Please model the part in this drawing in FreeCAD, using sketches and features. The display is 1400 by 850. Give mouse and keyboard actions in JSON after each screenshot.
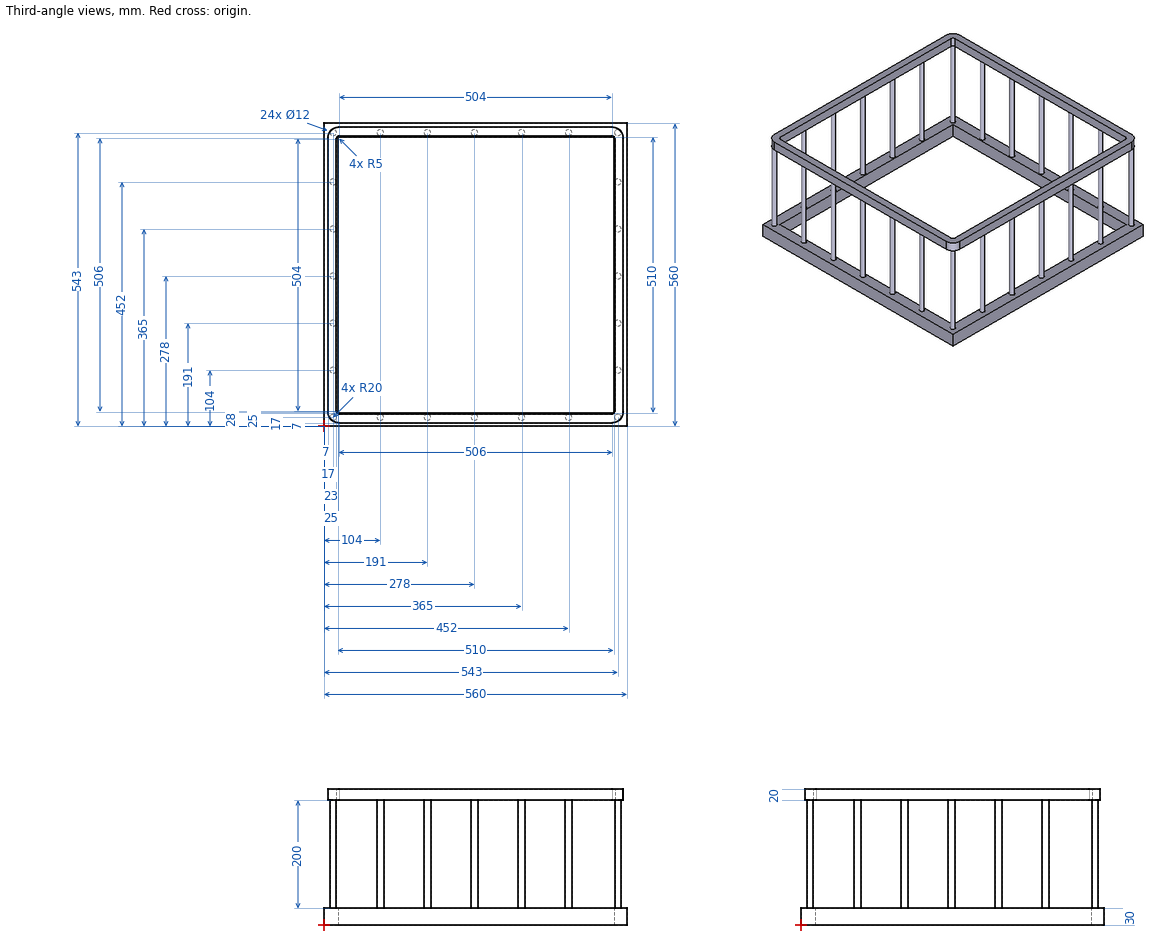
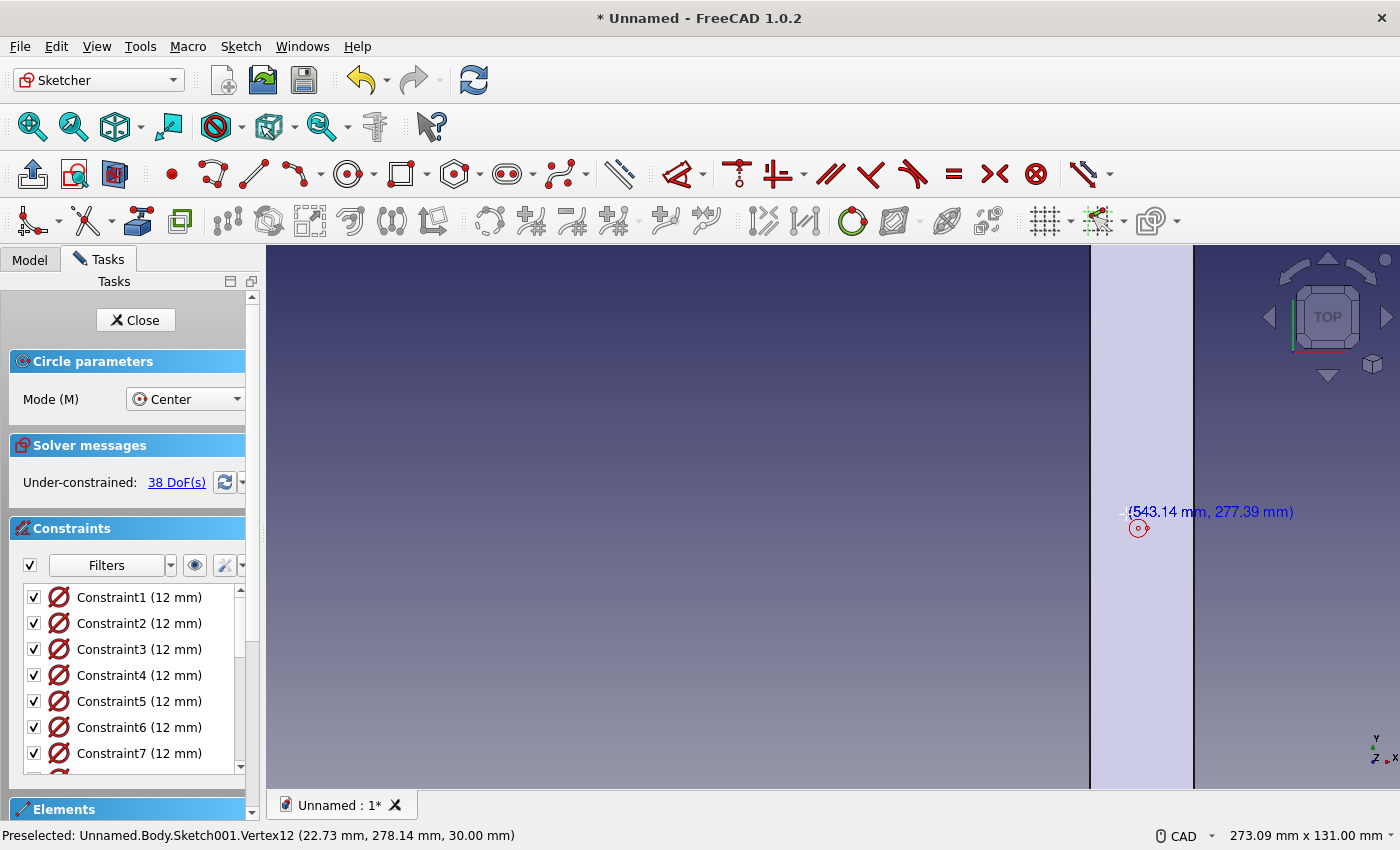
{"action": "scroll", "coordinate": [914, 515], "scroll_direction": "down", "scroll_amount": 9}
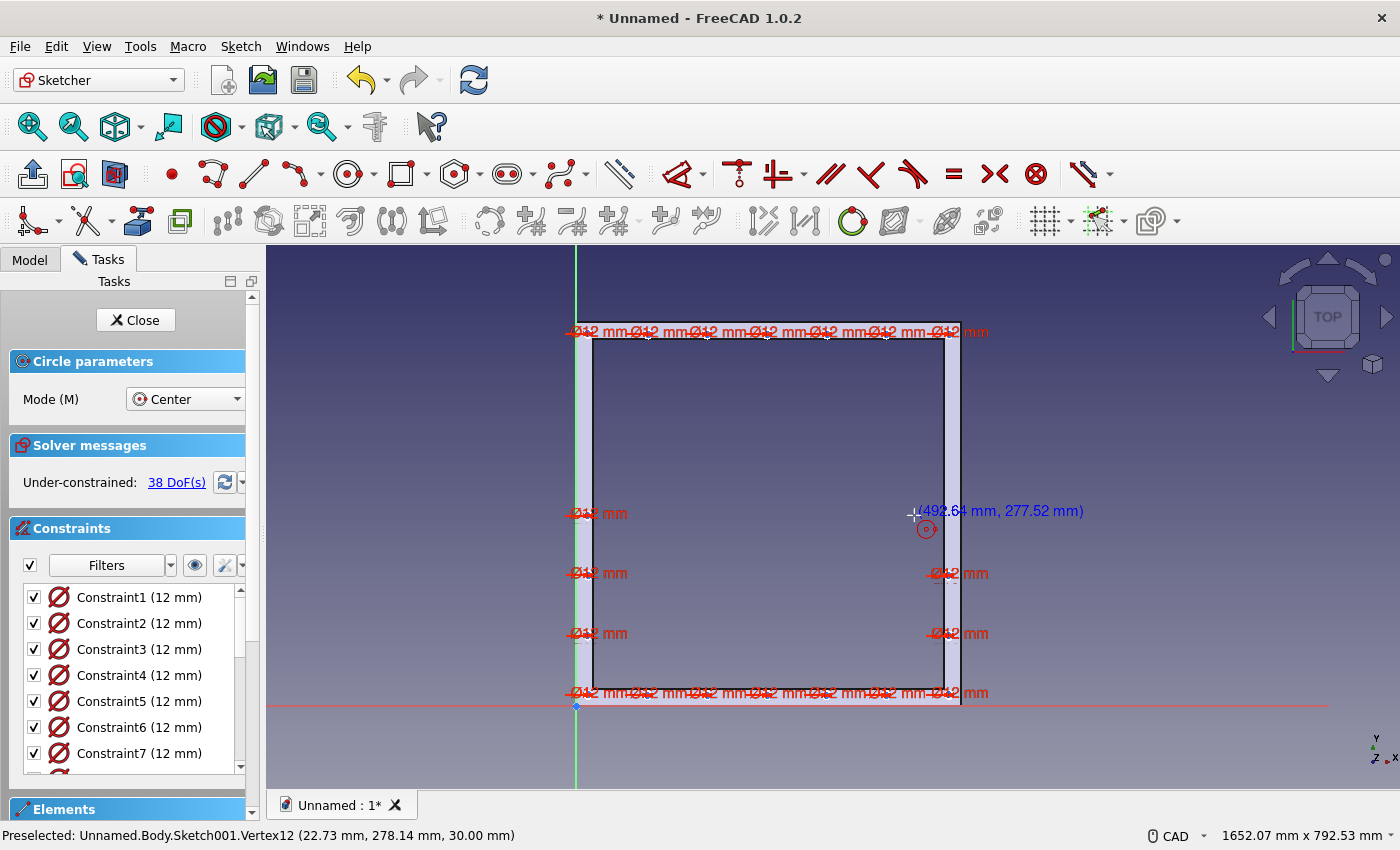
{"action": "left_click", "coordinate": [949, 515]}
{"action": "mouse_move", "coordinate": [952, 512]}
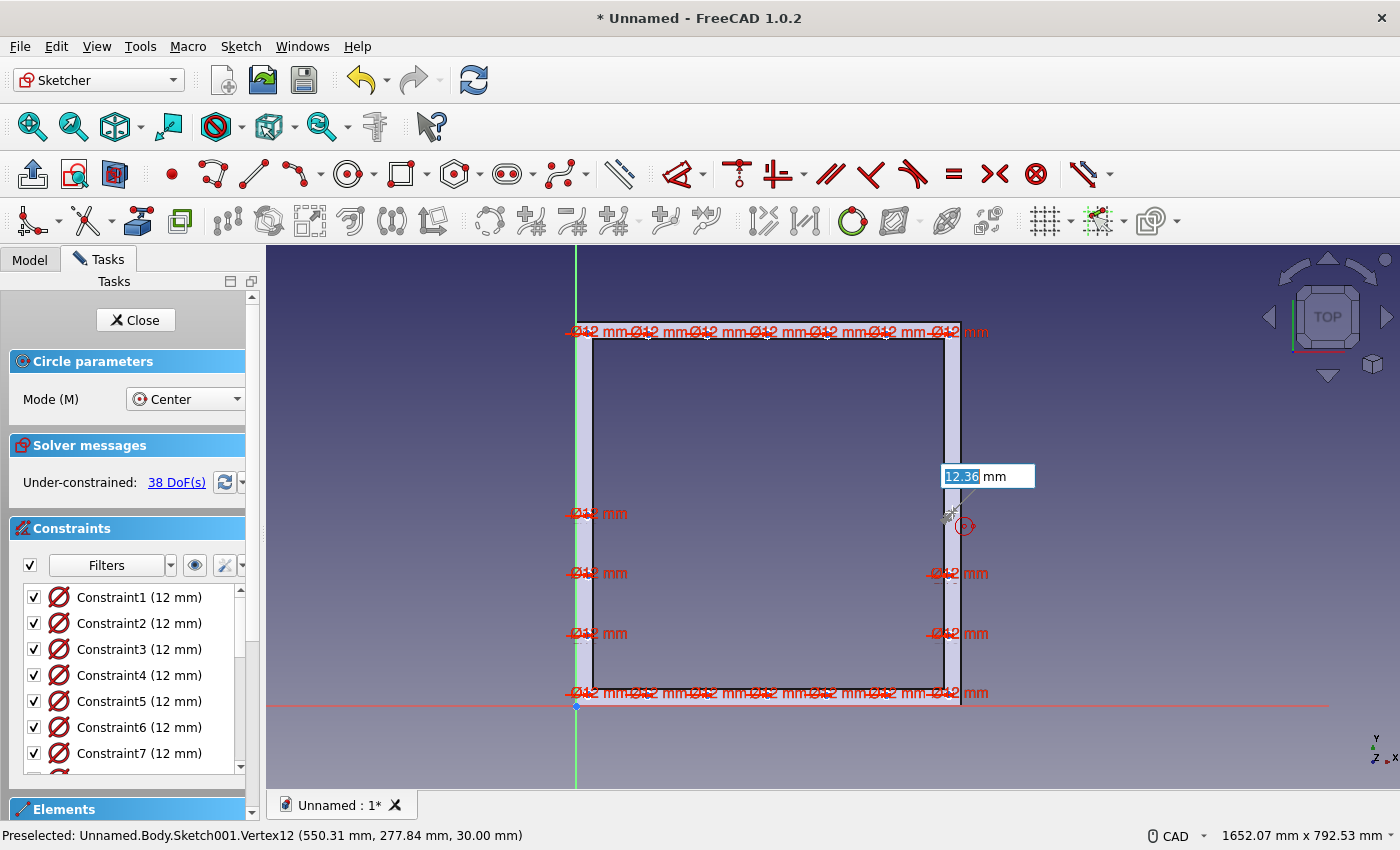
{"action": "type", "text": "12"}
{"action": "key", "text": "Return"}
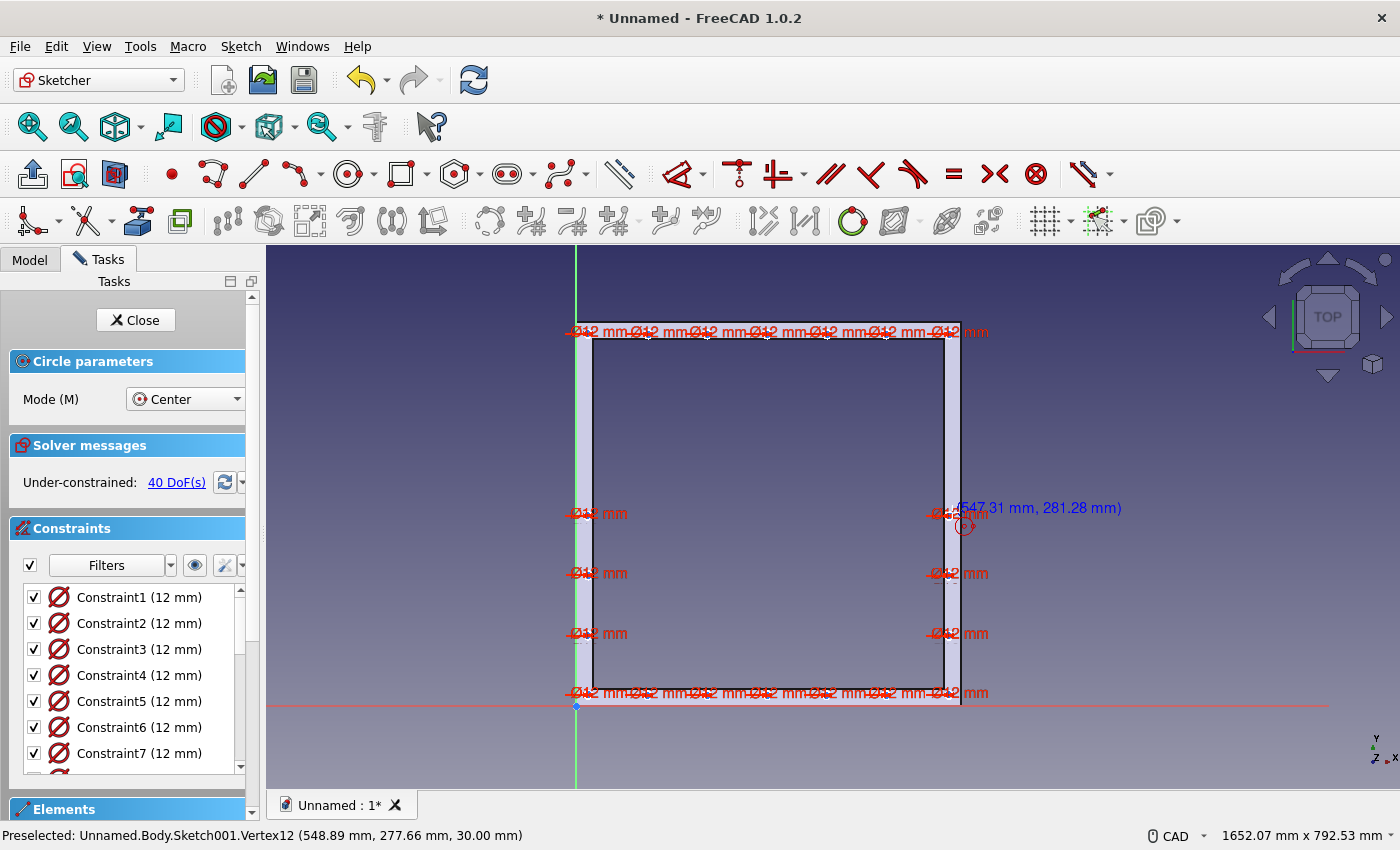
{"action": "scroll", "coordinate": [588, 456], "scroll_direction": "up", "scroll_amount": 9}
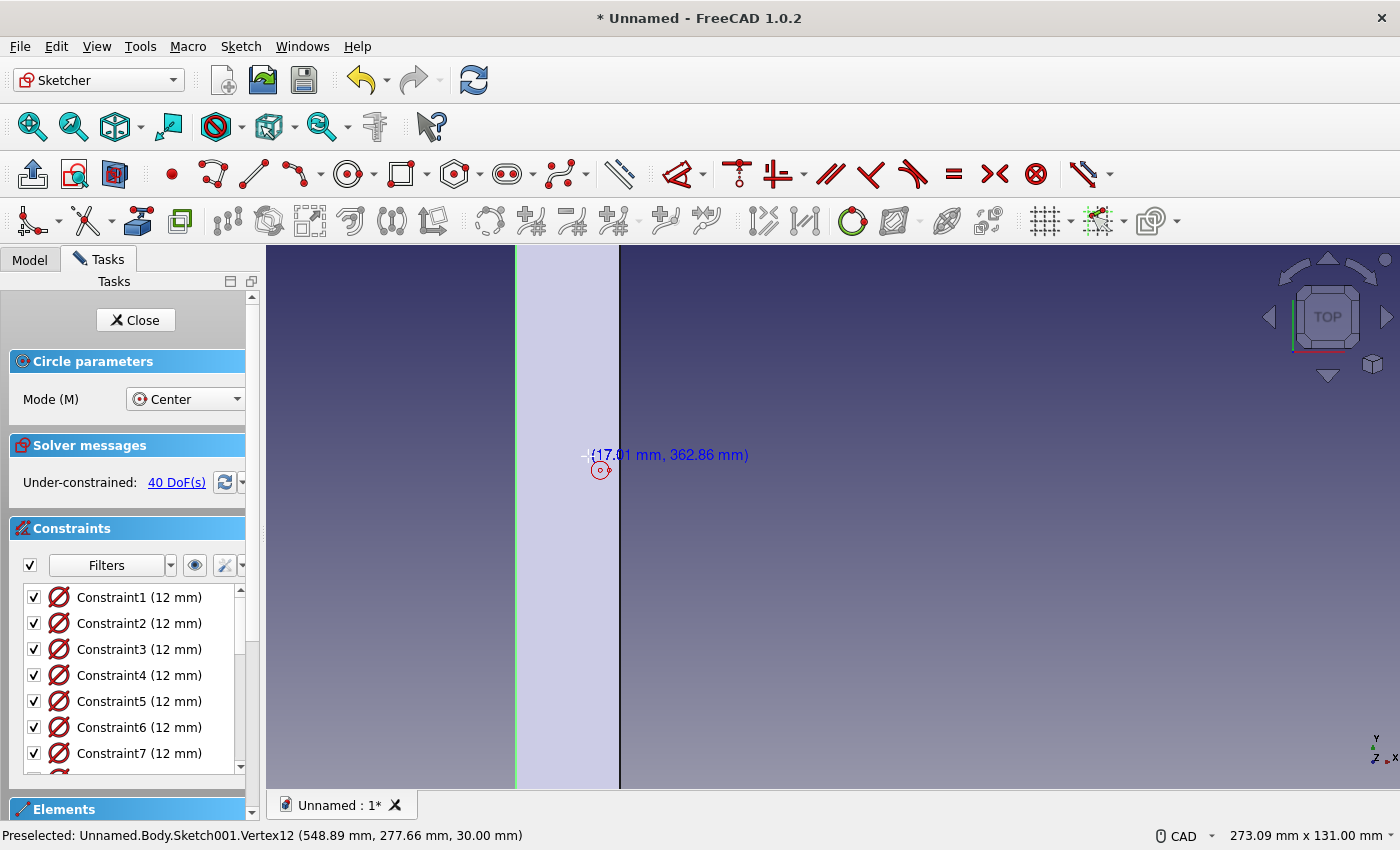
{"action": "scroll", "coordinate": [588, 456], "scroll_direction": "down", "scroll_amount": 9}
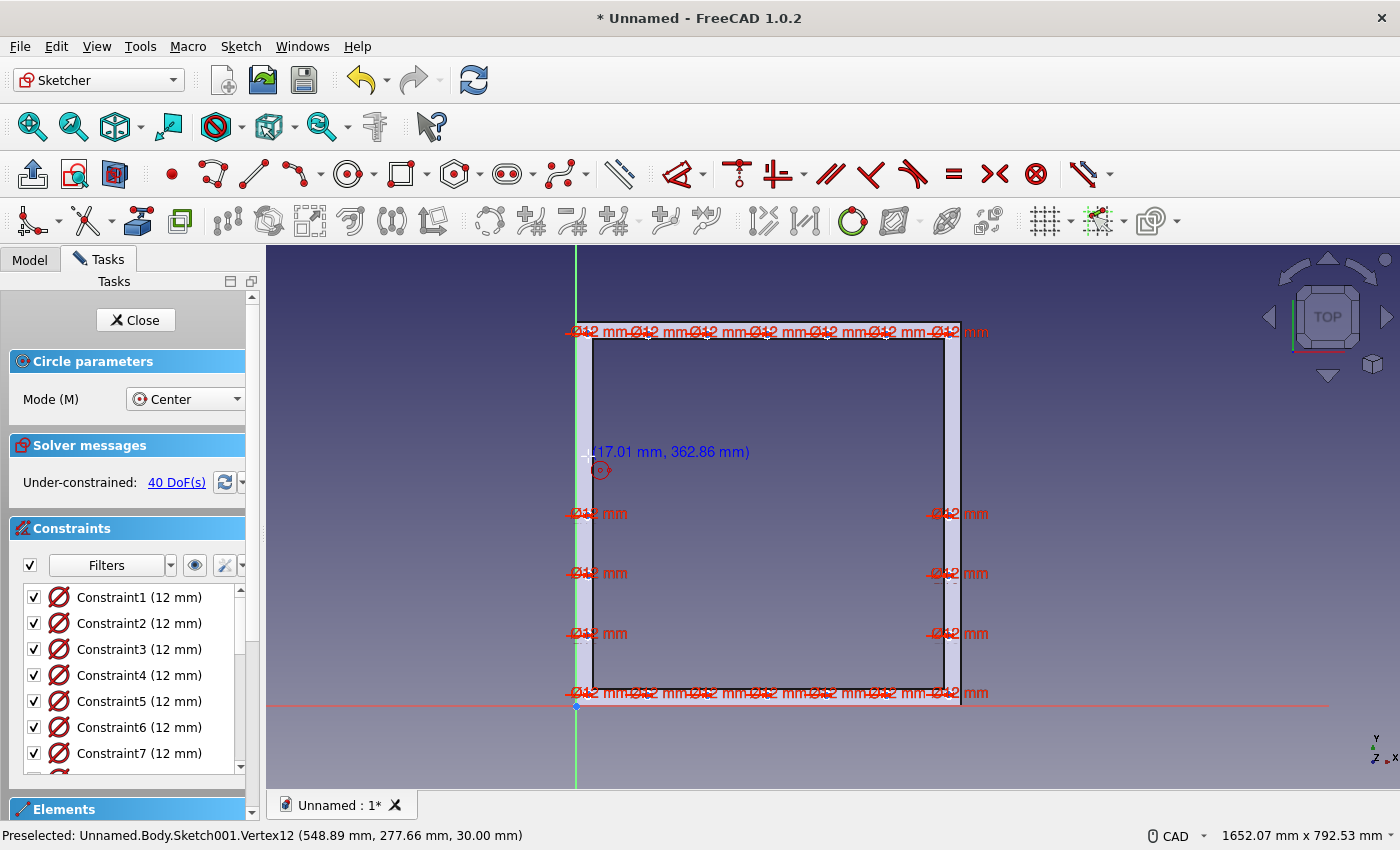
{"action": "scroll", "coordinate": [588, 456], "scroll_direction": "up", "scroll_amount": 2}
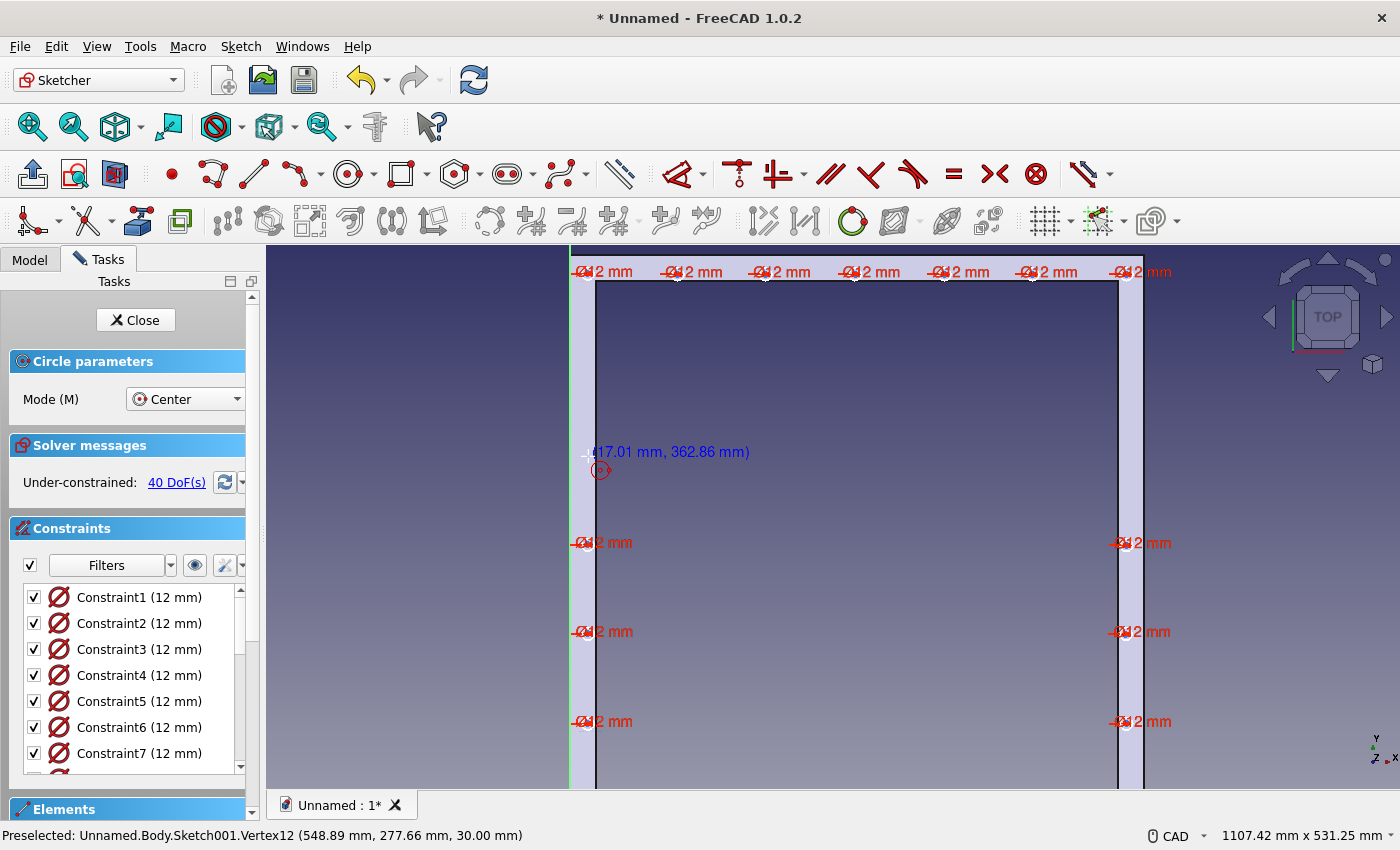
{"action": "left_click", "coordinate": [588, 455]}
{"action": "mouse_move", "coordinate": [592, 451]}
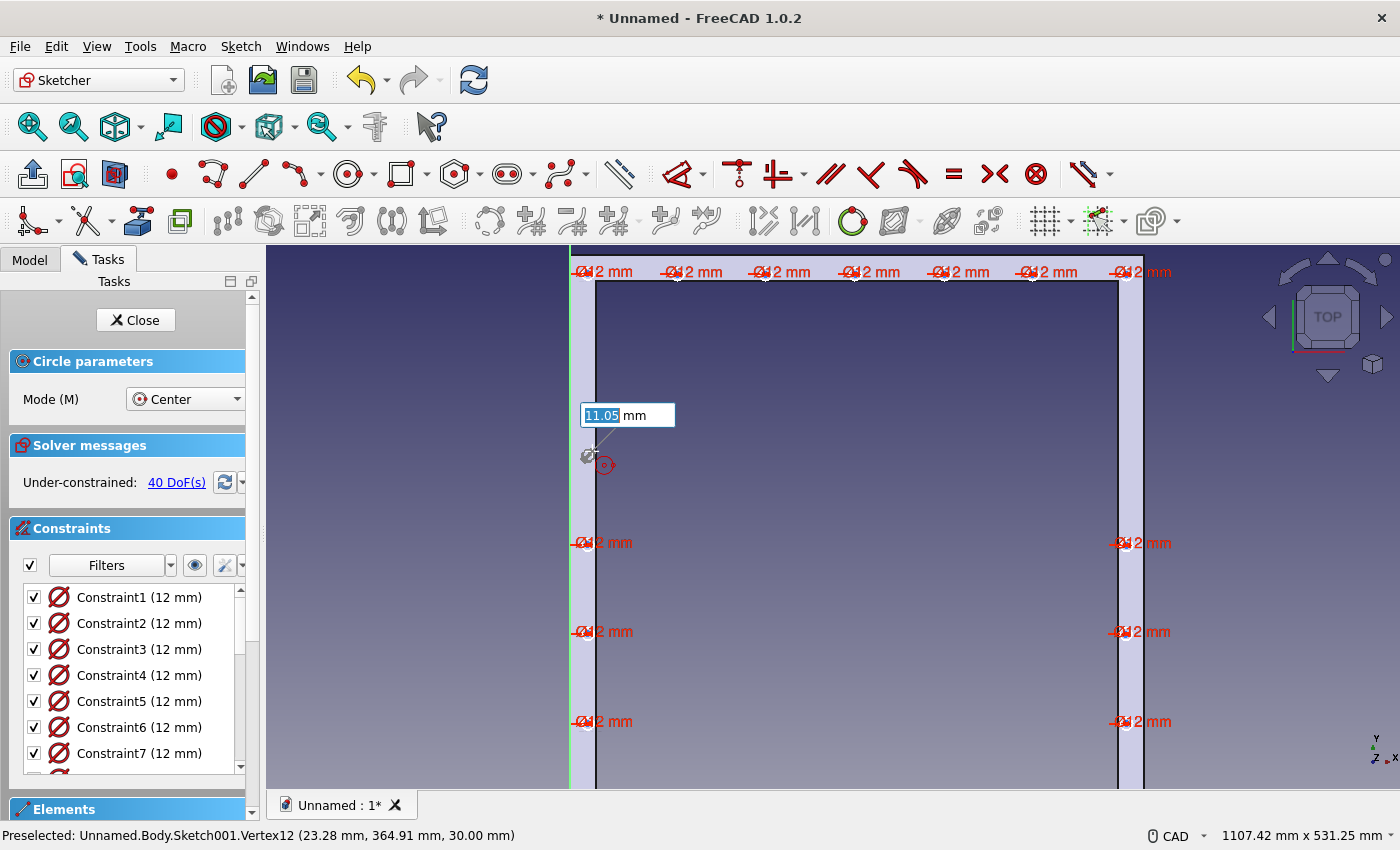
{"action": "type", "text": "12"}
{"action": "key", "text": "Return"}